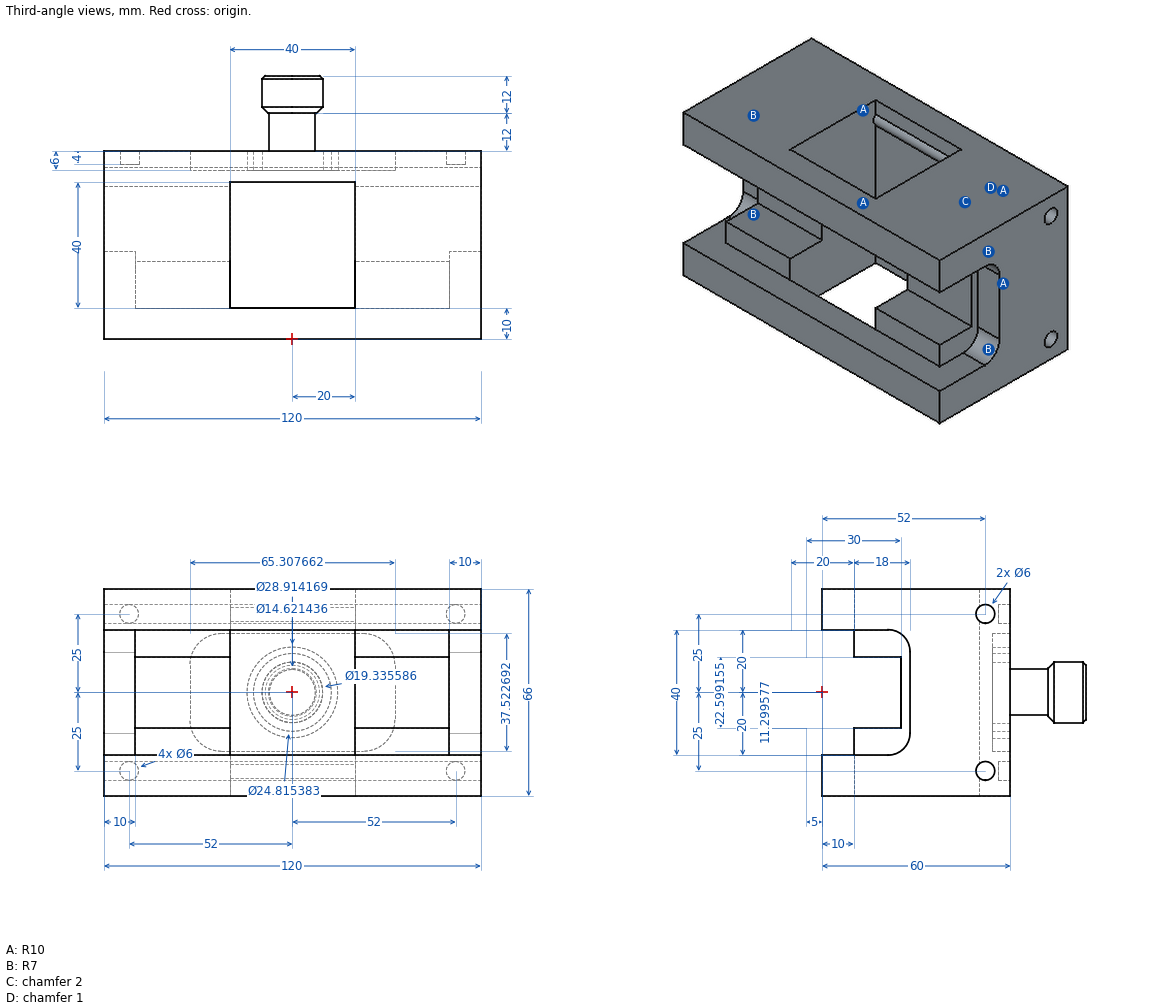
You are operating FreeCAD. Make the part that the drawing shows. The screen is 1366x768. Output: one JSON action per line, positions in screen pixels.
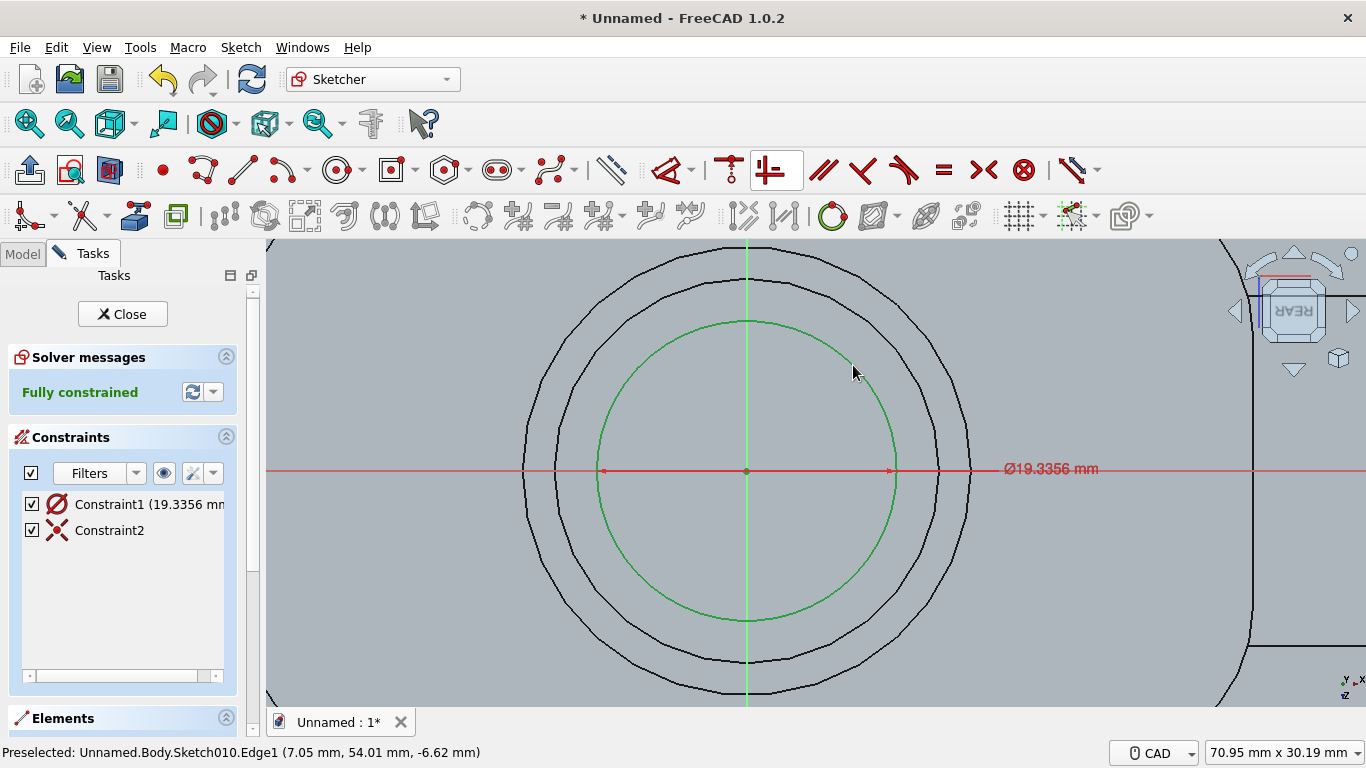
{"action": "left_click", "coordinate": [123, 314]}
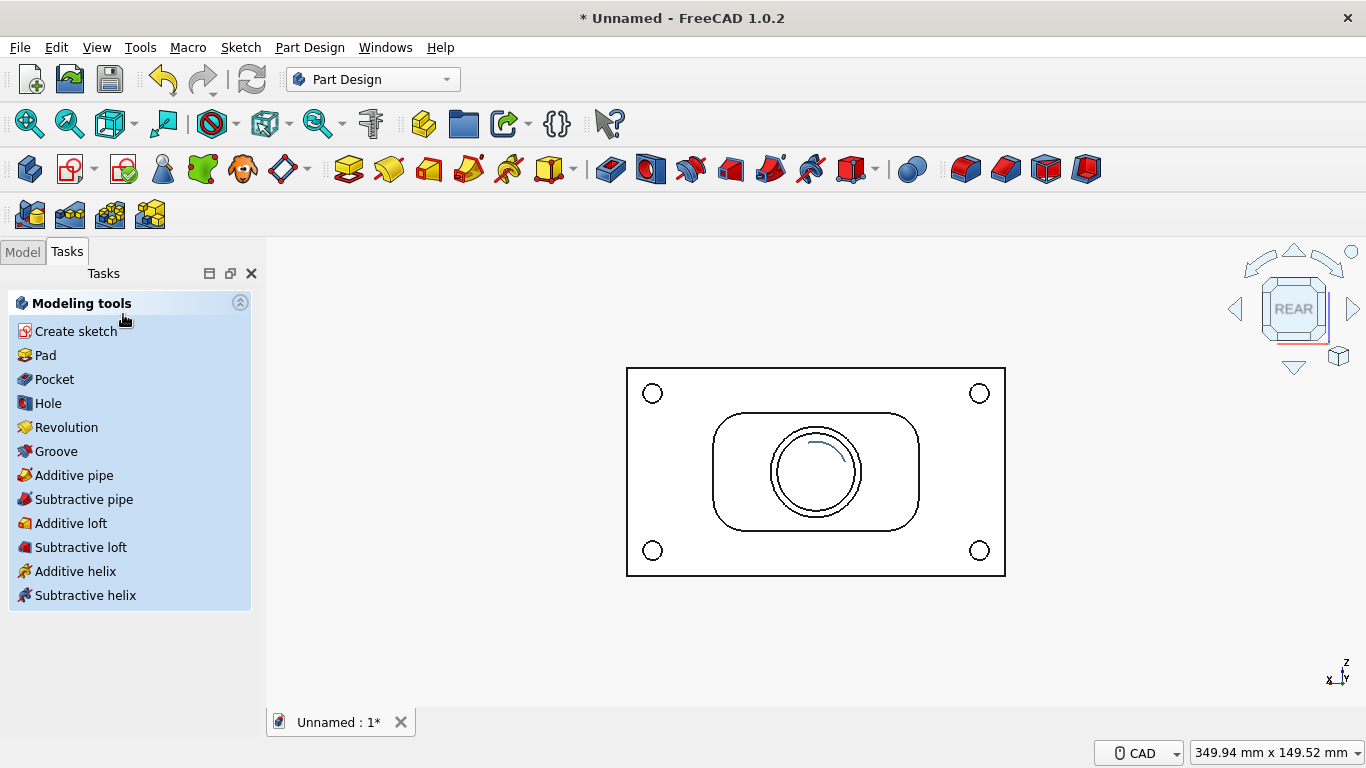
{"action": "left_click", "coordinate": [350, 170]}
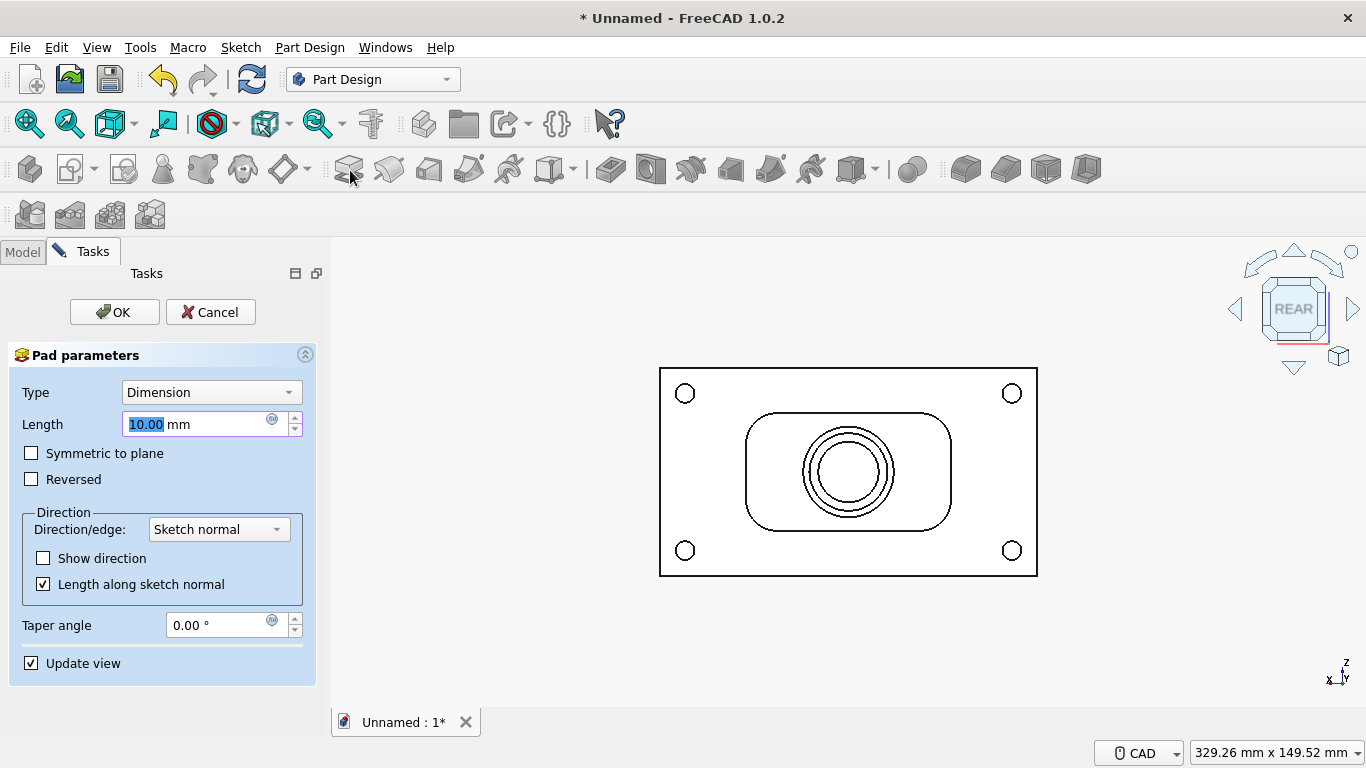
{"action": "type", "text": "6"}
{"action": "key", "text": "Tab"}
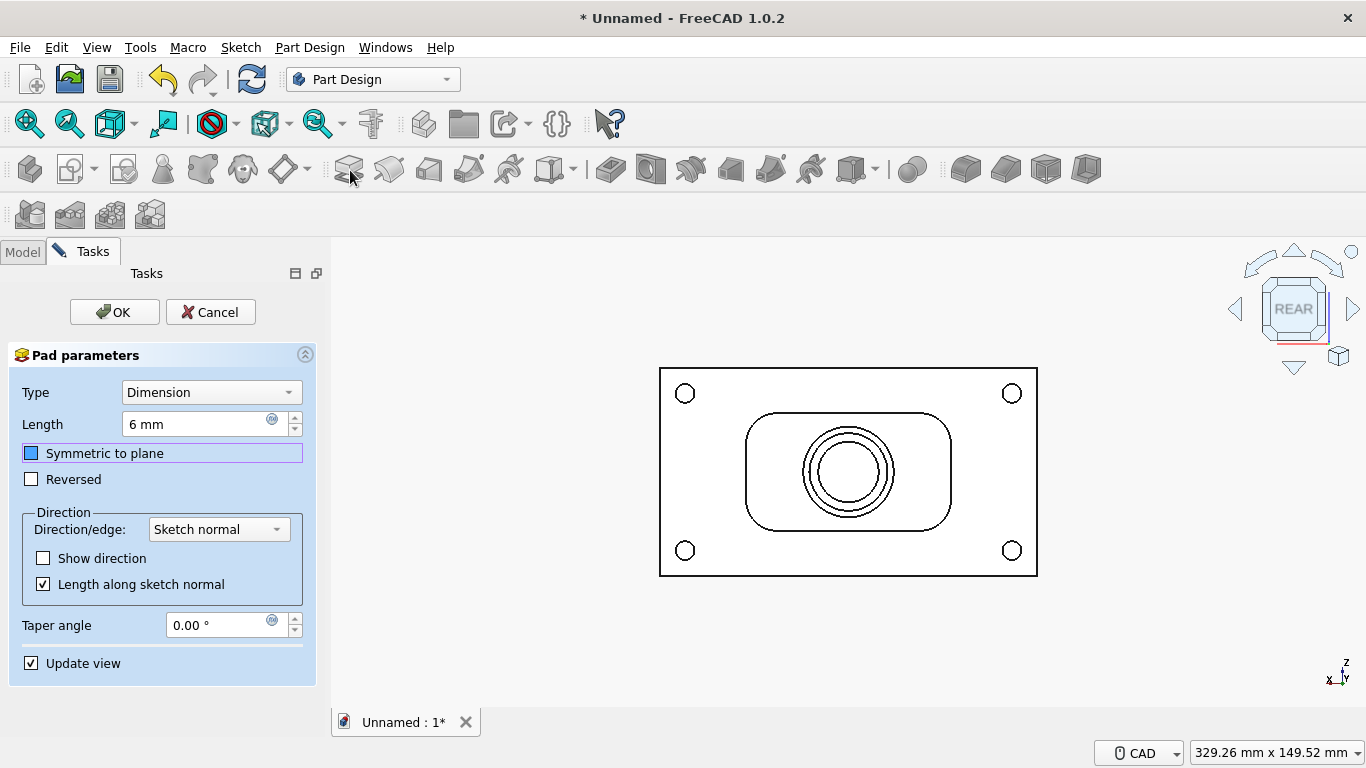
{"action": "left_click", "coordinate": [115, 312]}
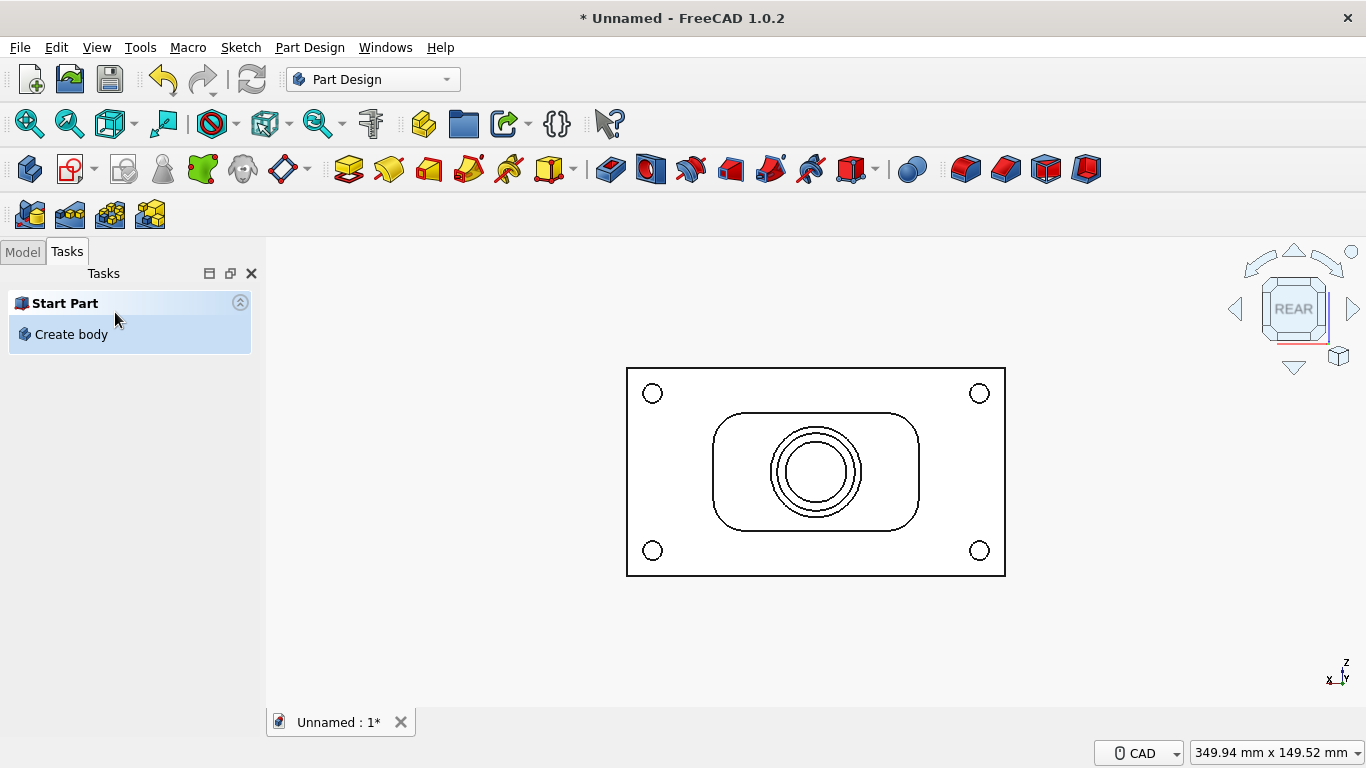
{"action": "left_click", "coordinate": [30, 124]}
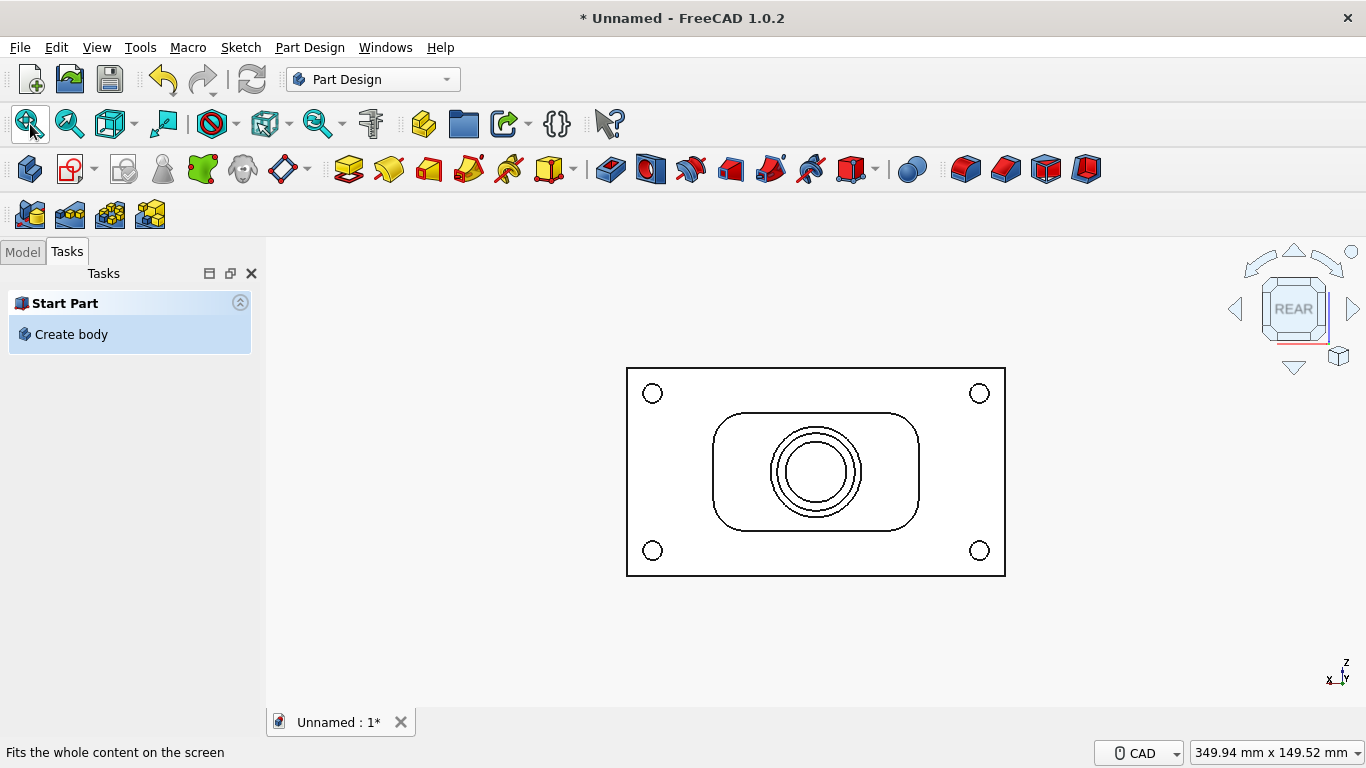
{"action": "left_click", "coordinate": [654, 441]}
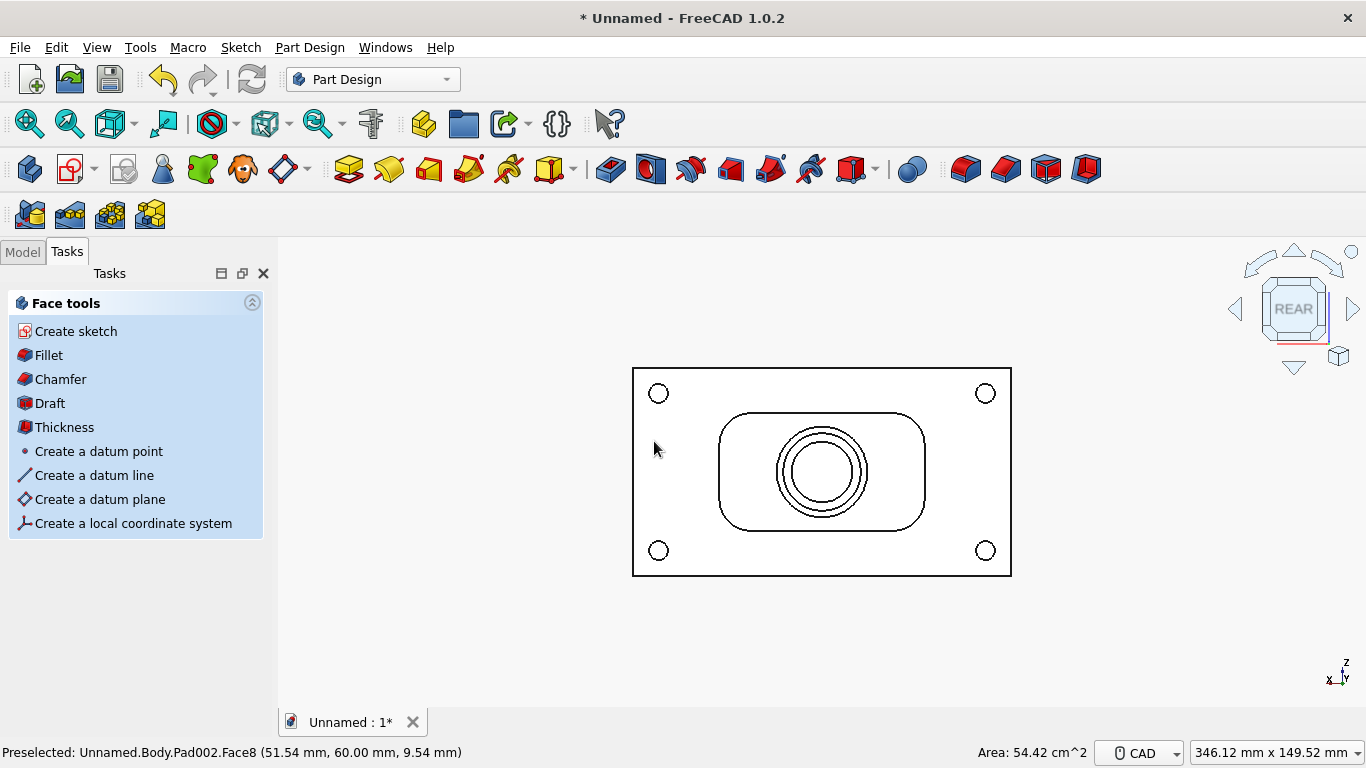
{"action": "left_click", "coordinate": [70, 170]}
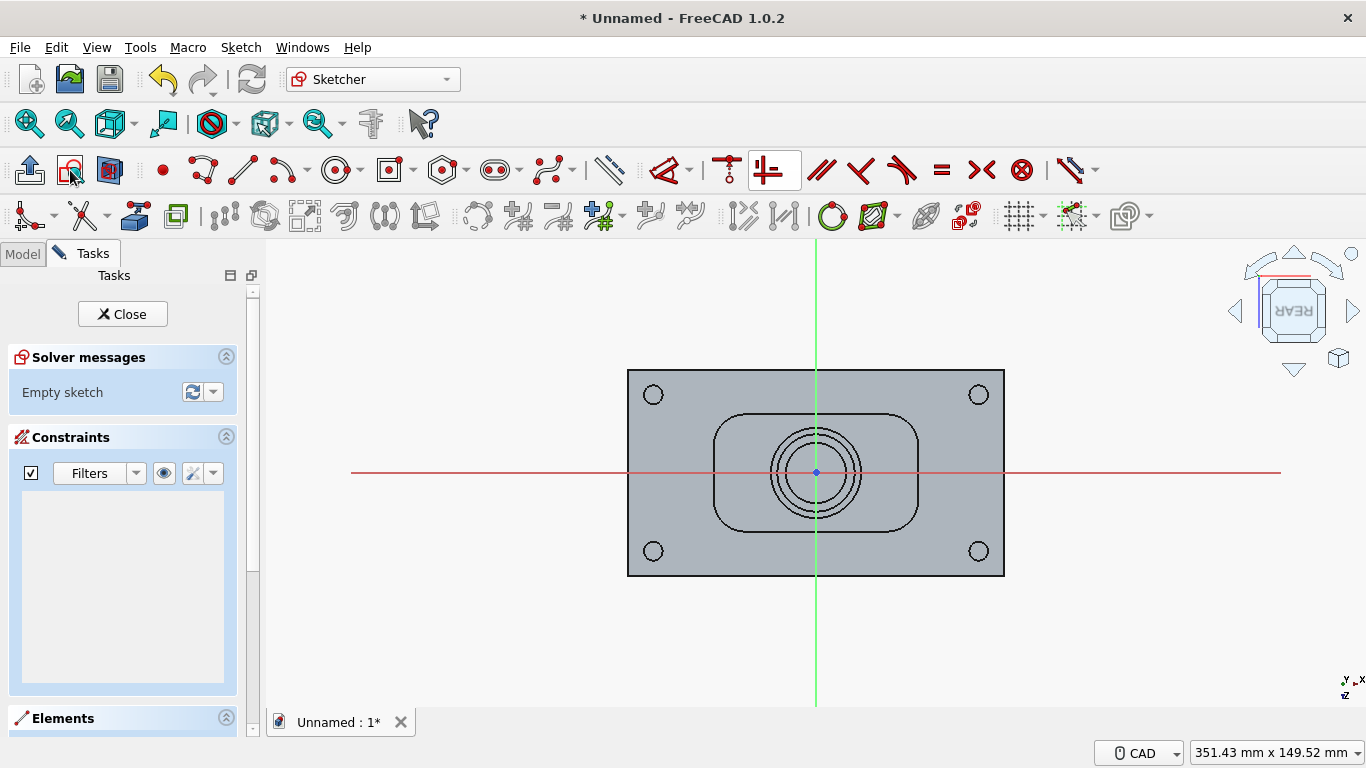
{"action": "scroll", "coordinate": [830, 473], "scroll_direction": "up", "scroll_amount": 9}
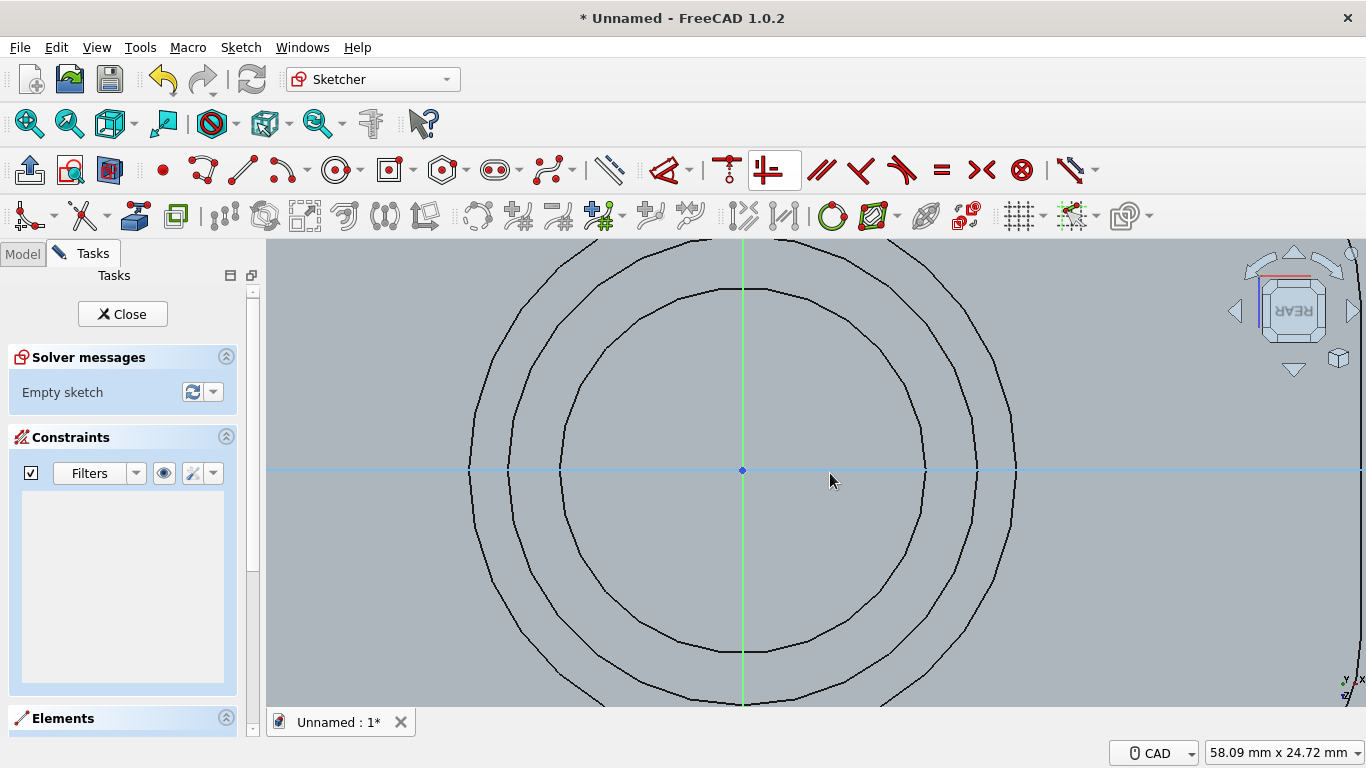
{"action": "left_click", "coordinate": [336, 170]}